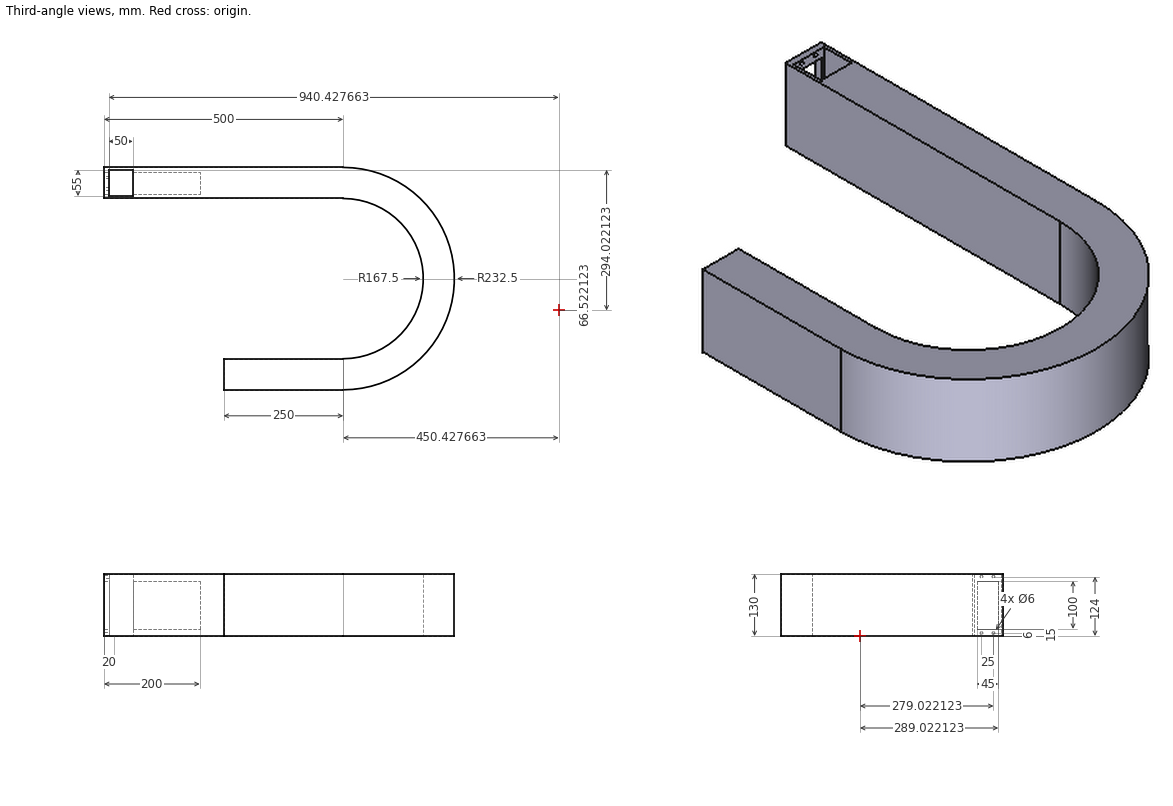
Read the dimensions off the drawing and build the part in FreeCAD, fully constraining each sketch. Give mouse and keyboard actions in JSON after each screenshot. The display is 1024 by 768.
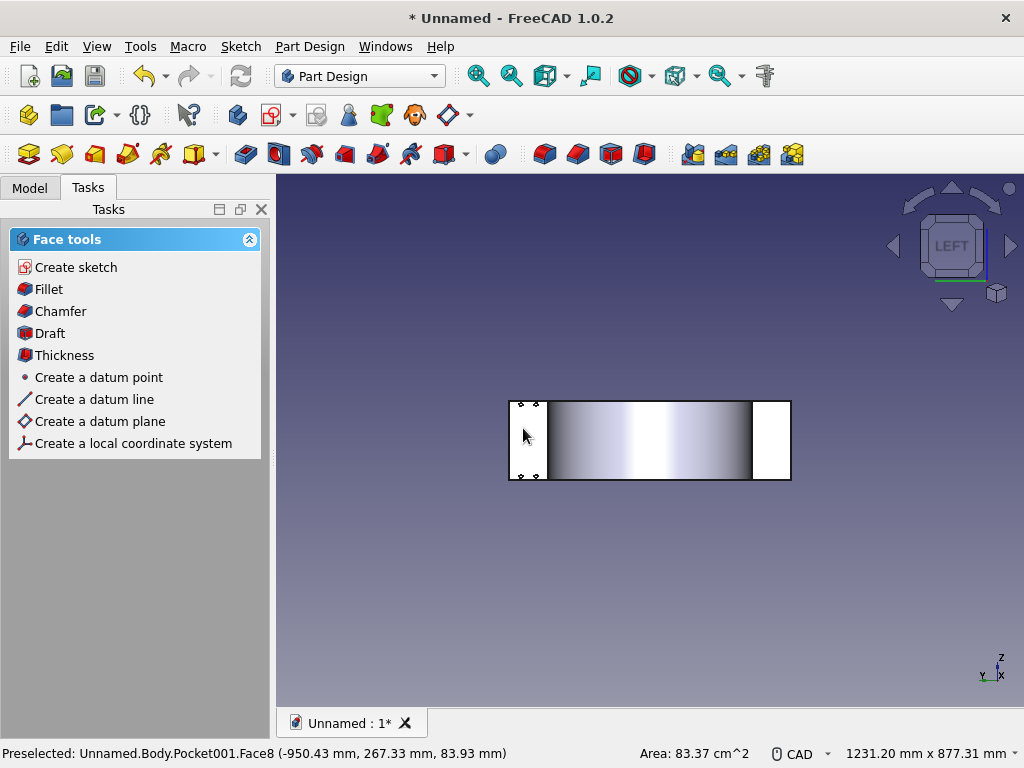
{"action": "left_click", "coordinate": [270, 116]}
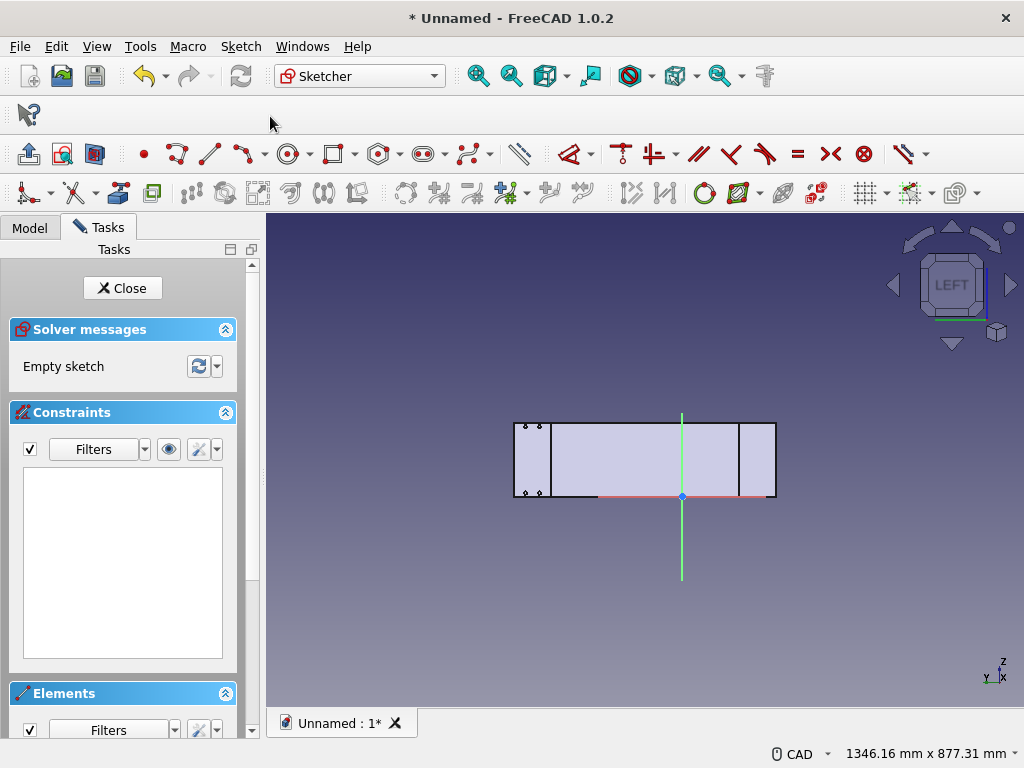
{"action": "scroll", "coordinate": [524, 460], "scroll_direction": "up", "scroll_amount": 9}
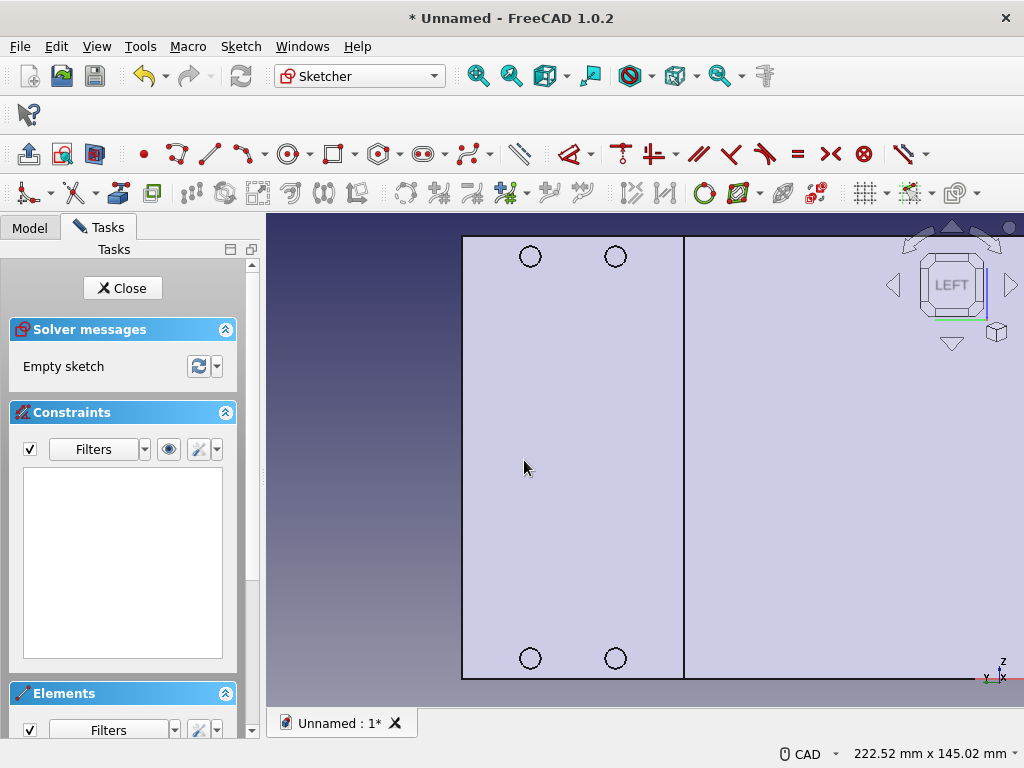
{"action": "key", "text": "g r"}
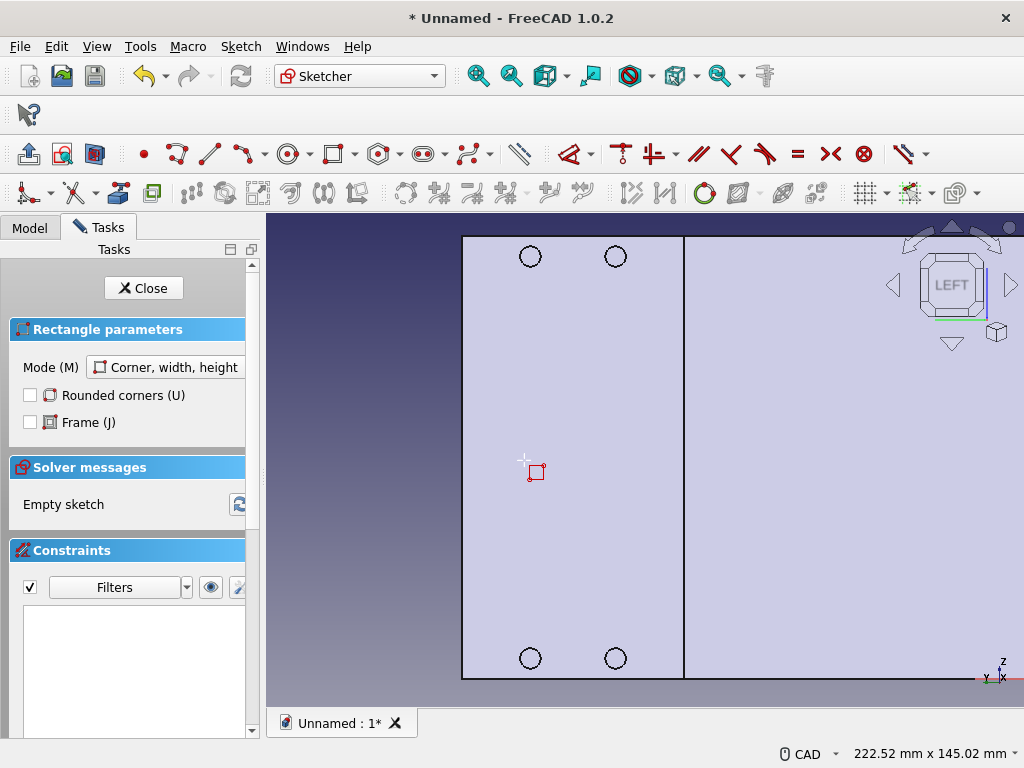
{"action": "left_click", "coordinate": [496, 287]}
{"action": "mouse_move", "coordinate": [650, 628]}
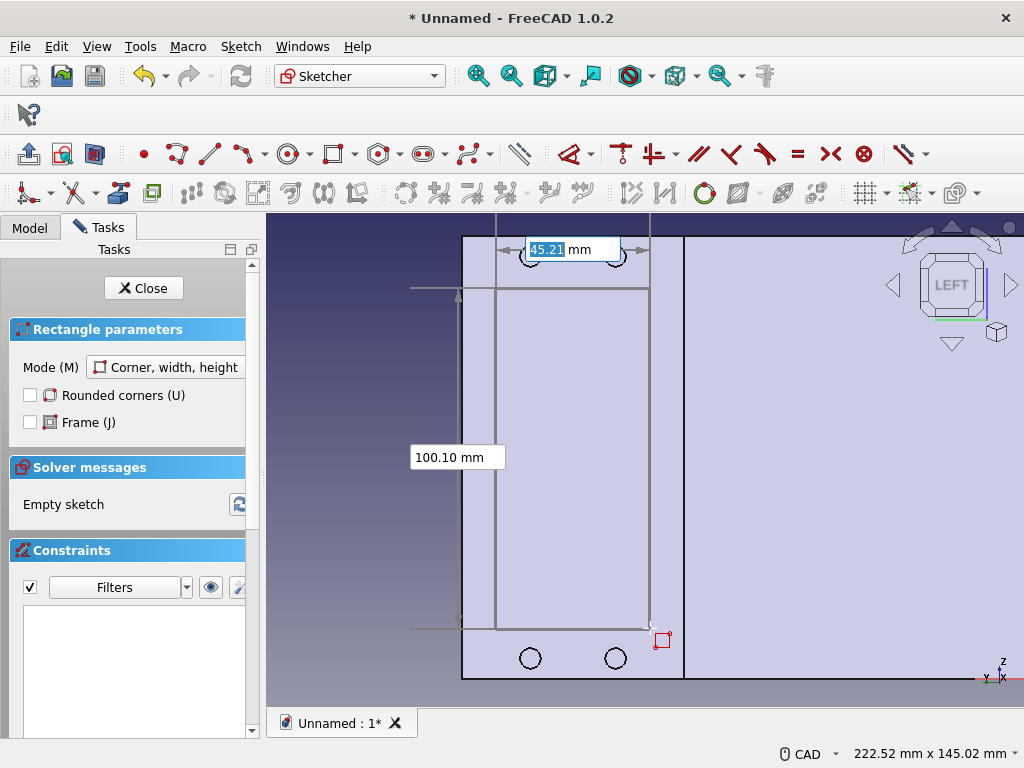
{"action": "type", "text": "45"}
{"action": "key", "text": "Tab"}
{"action": "type", "text": "100"}
{"action": "key", "text": "Return"}
{"action": "key", "text": "Escape"}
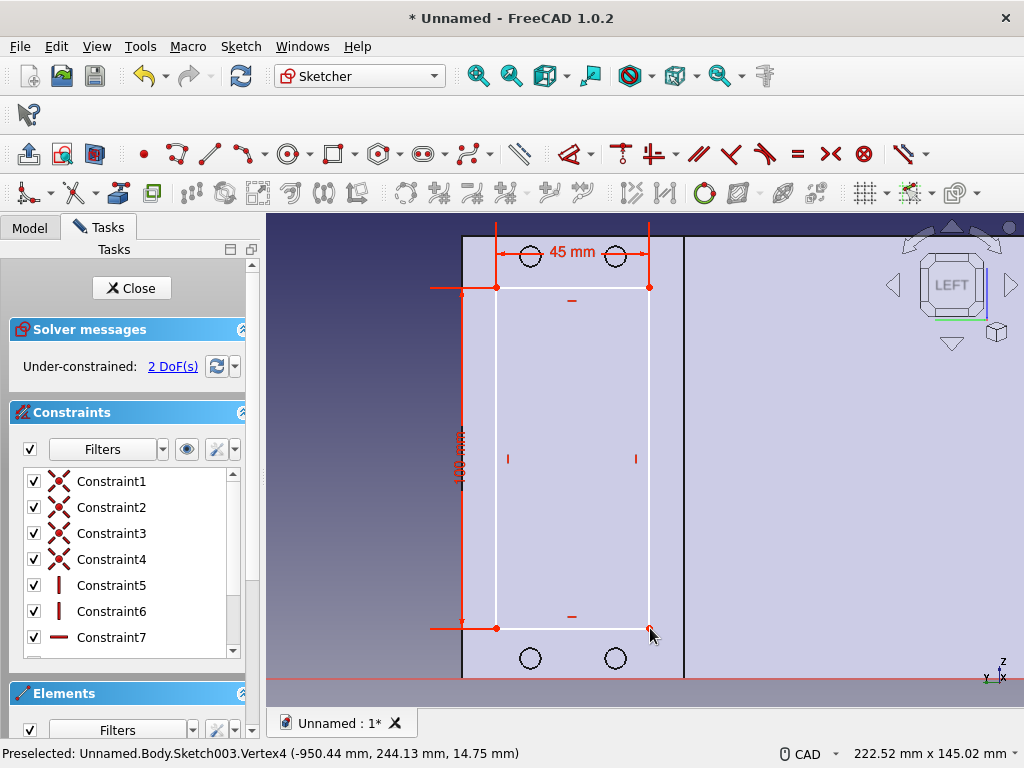
{"action": "key", "text": "d"}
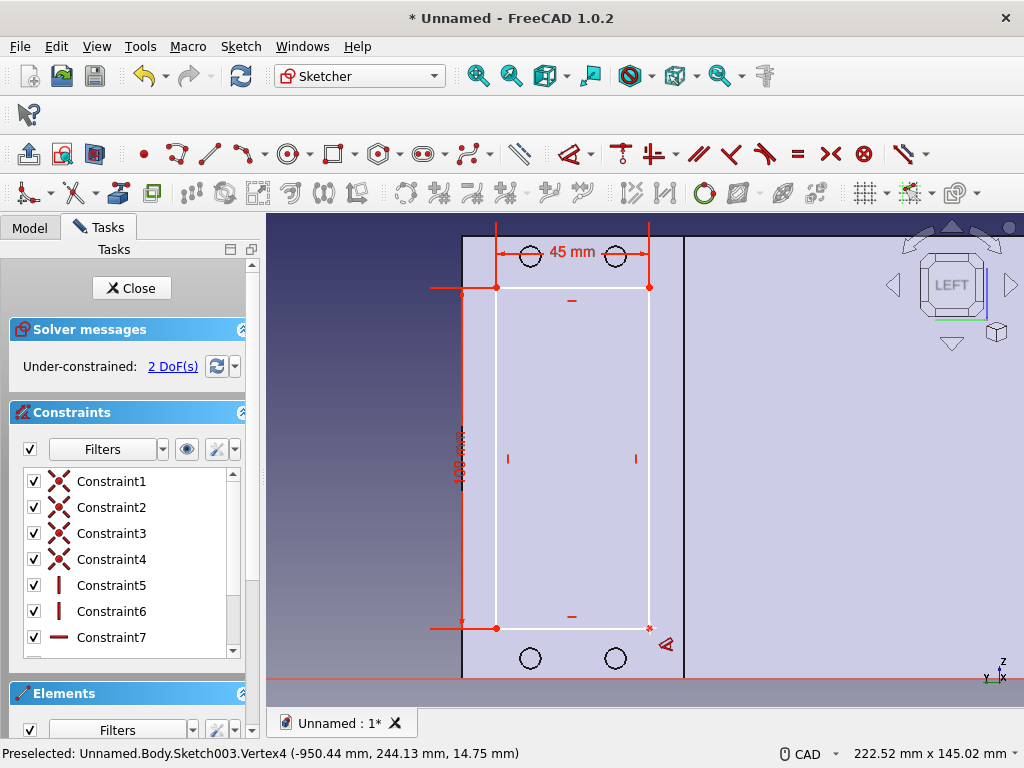
{"action": "left_click", "coordinate": [496, 629]}
{"action": "left_click", "coordinate": [462, 654]}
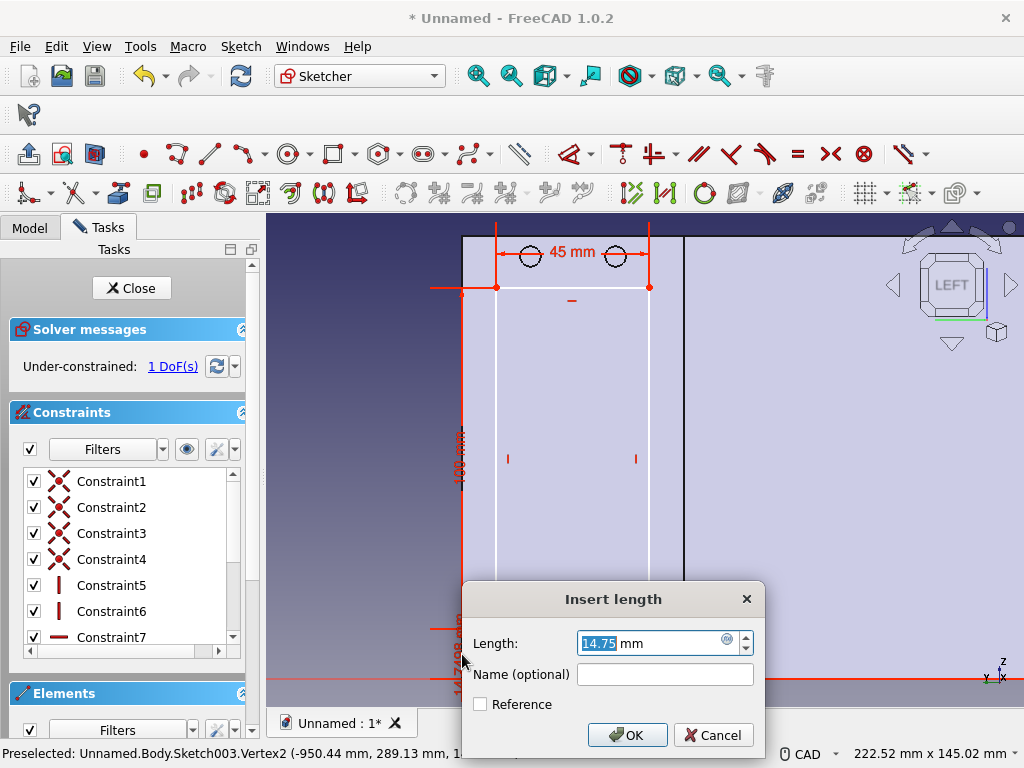
{"action": "type", "text": "15"}
{"action": "key", "text": "Return"}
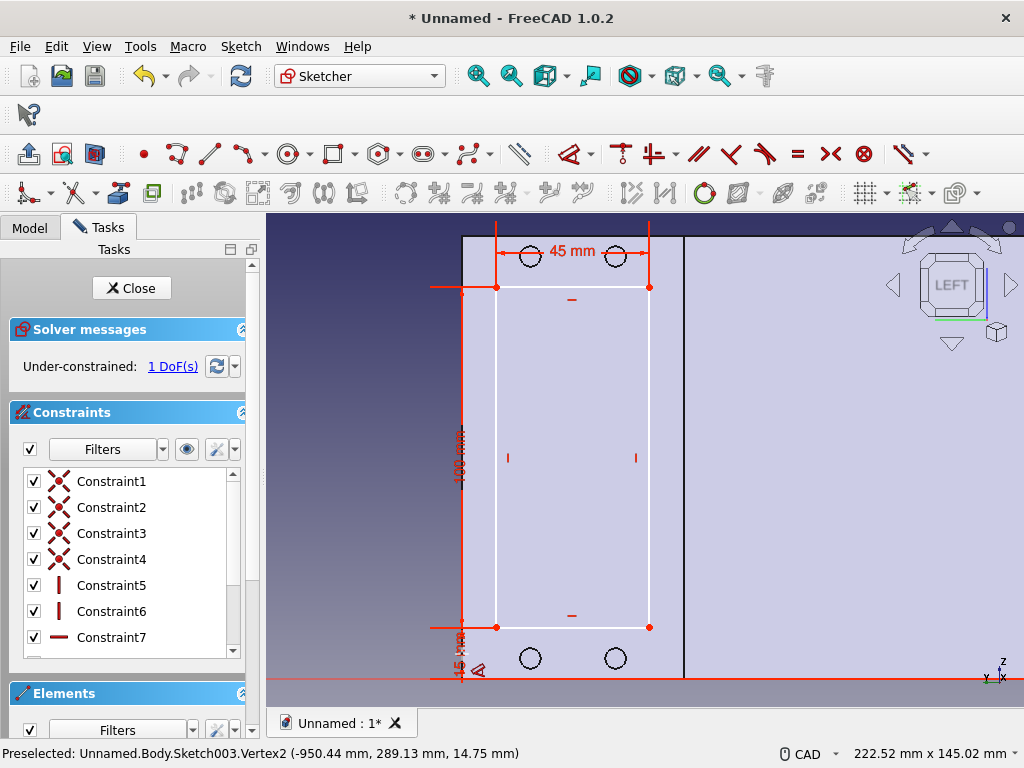
{"action": "left_click", "coordinate": [496, 287]}
{"action": "left_click", "coordinate": [678, 253]}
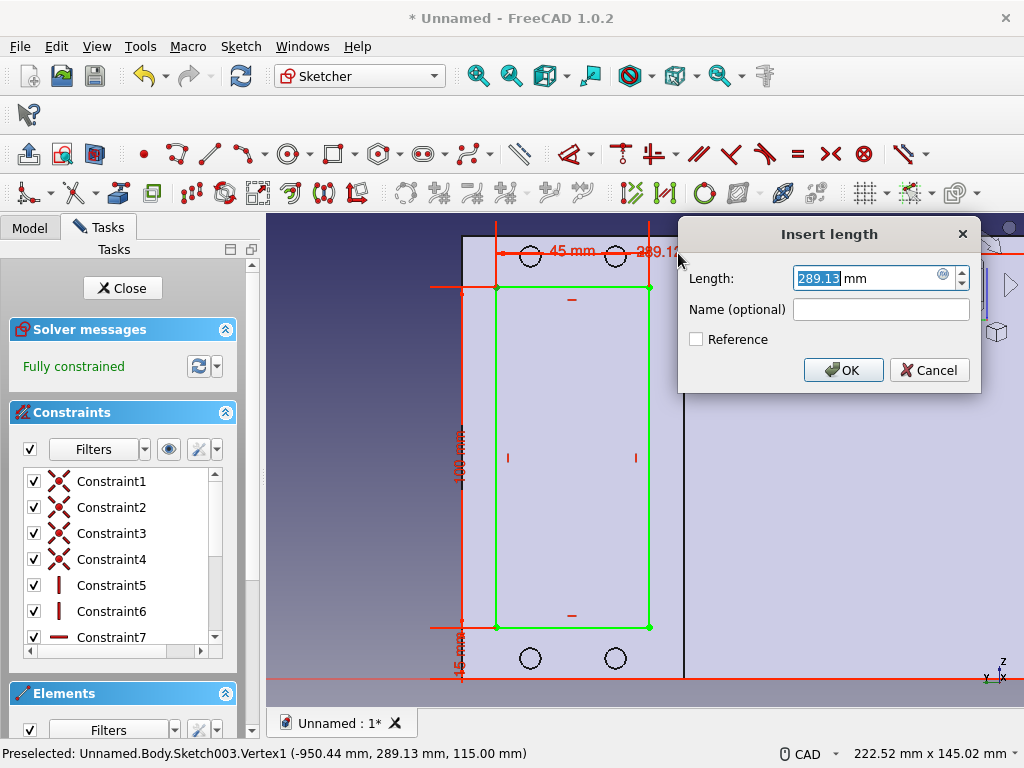
{"action": "type", "text": "289.022123"}
{"action": "key", "text": "Return"}
{"action": "key", "text": "Escape"}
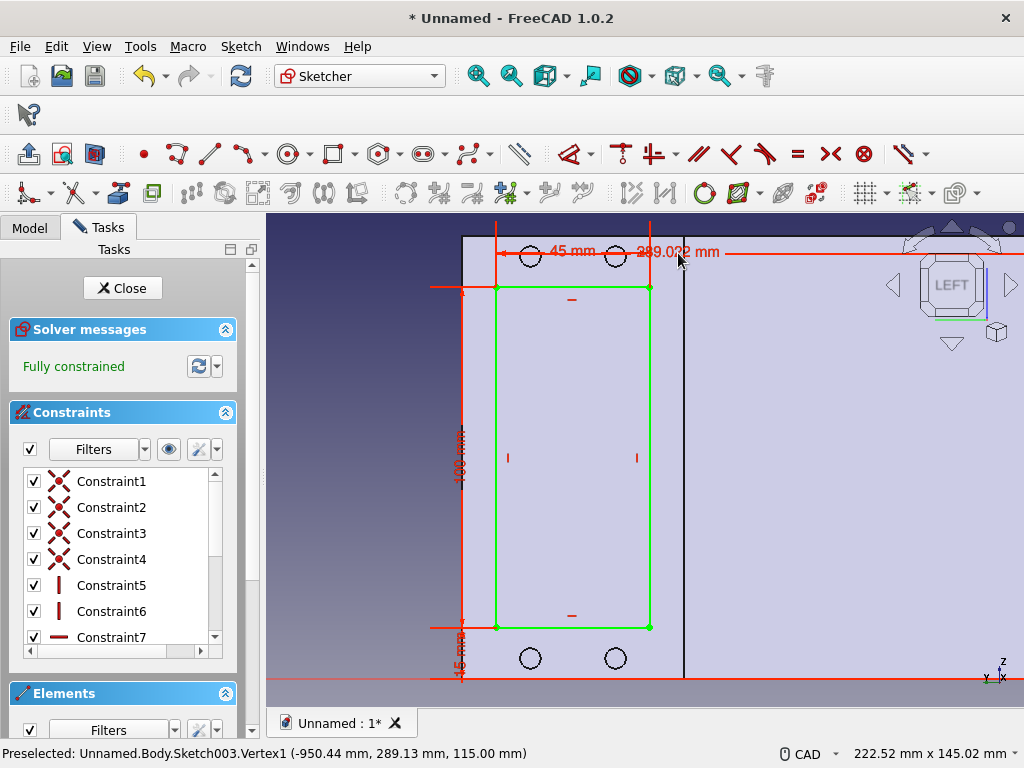
{"action": "left_click", "coordinate": [123, 288]}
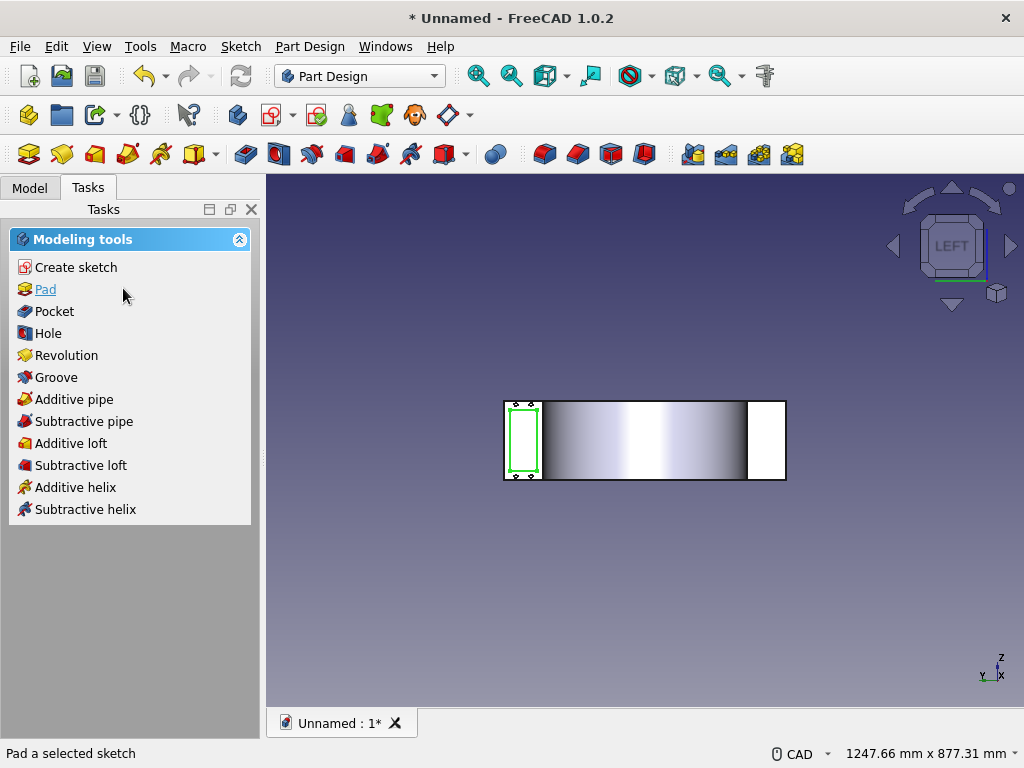
{"action": "left_click", "coordinate": [246, 154]}